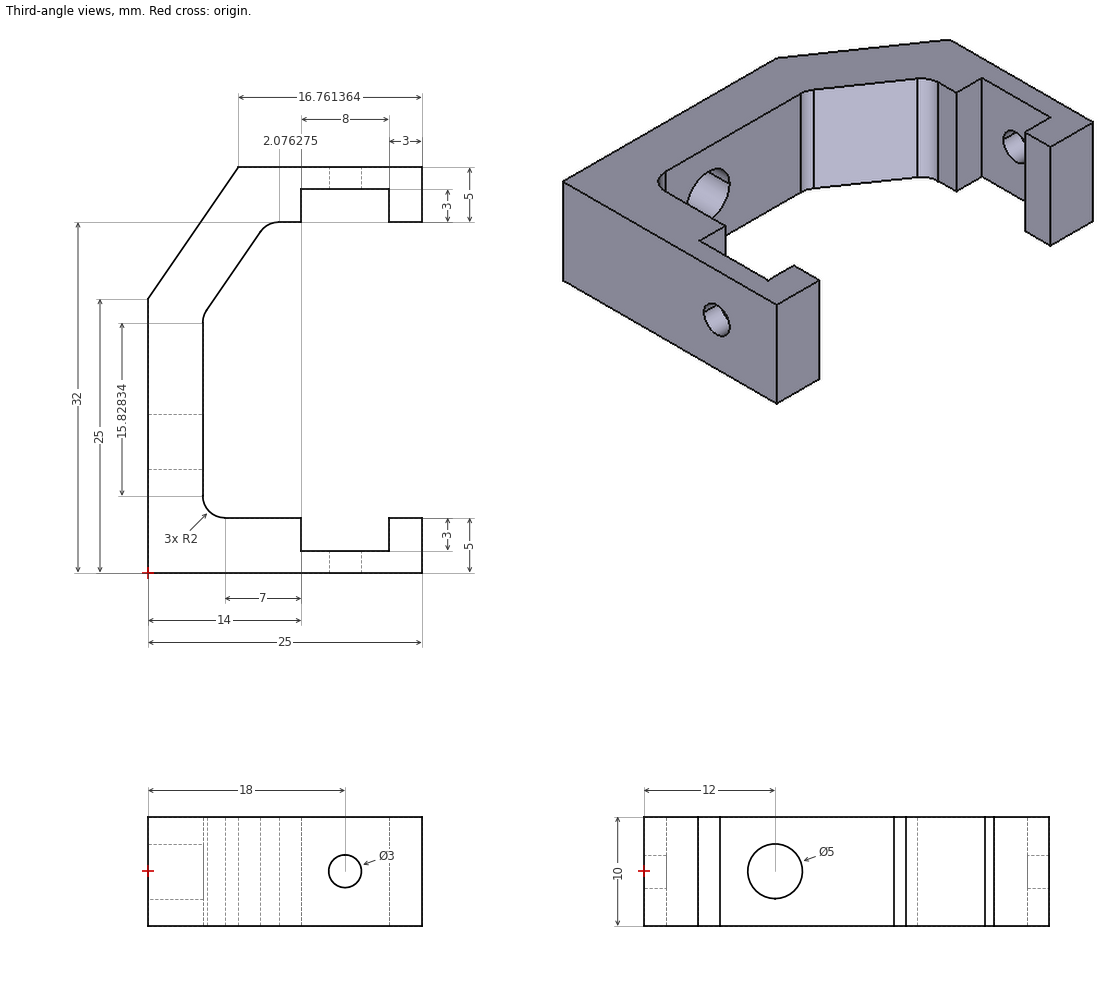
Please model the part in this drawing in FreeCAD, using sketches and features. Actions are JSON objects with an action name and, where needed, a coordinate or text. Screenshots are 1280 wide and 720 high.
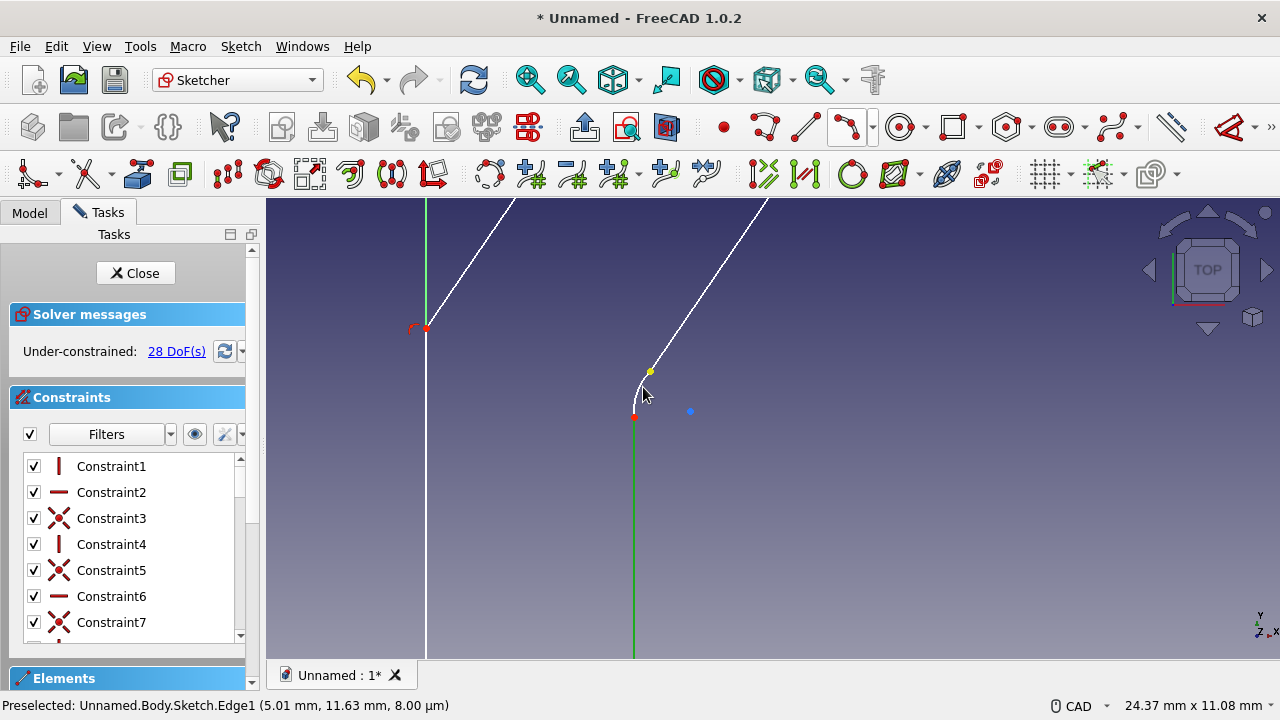
{"action": "left_click", "coordinate": [641, 384]}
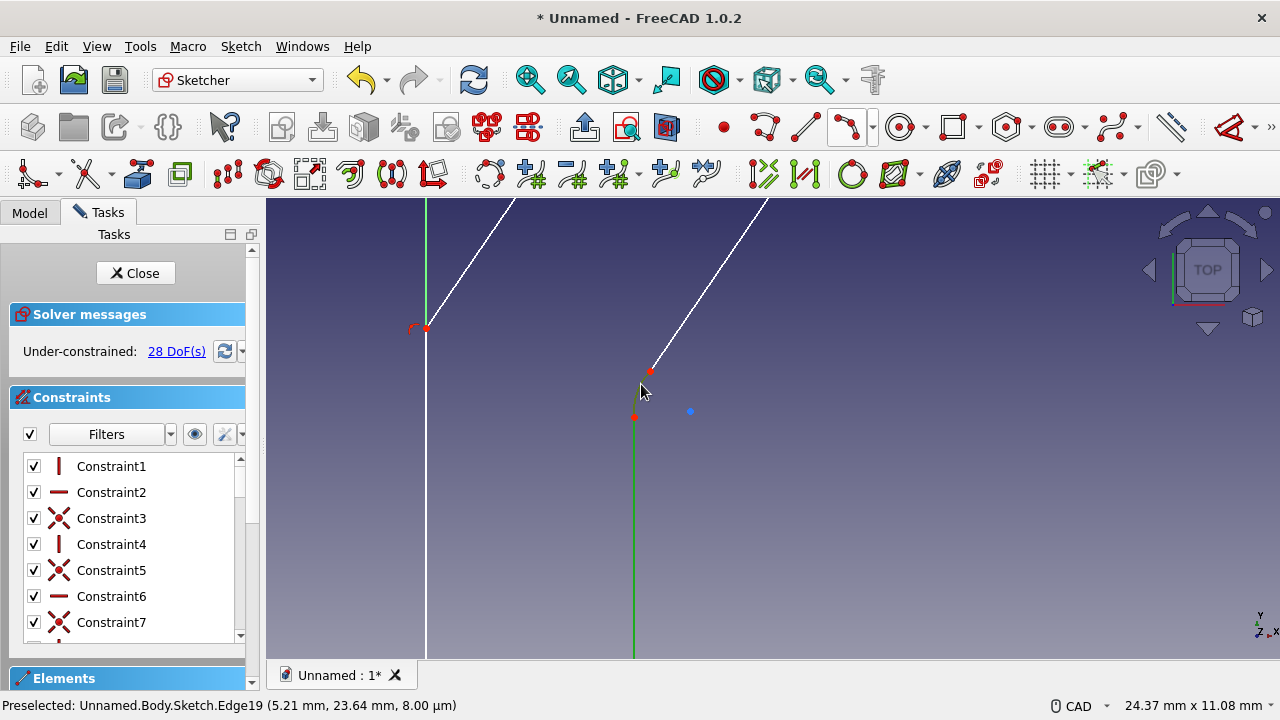
{"action": "key", "text": "t"}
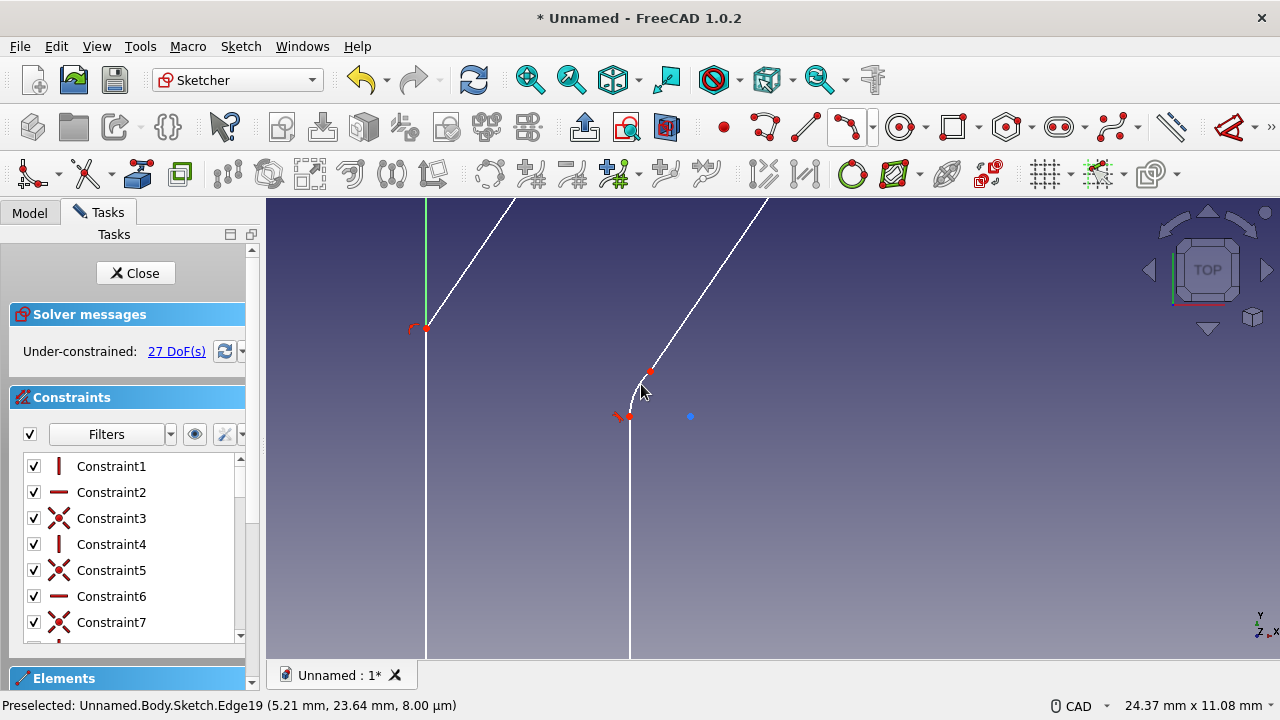
{"action": "scroll", "coordinate": [643, 386], "scroll_direction": "down", "scroll_amount": 8}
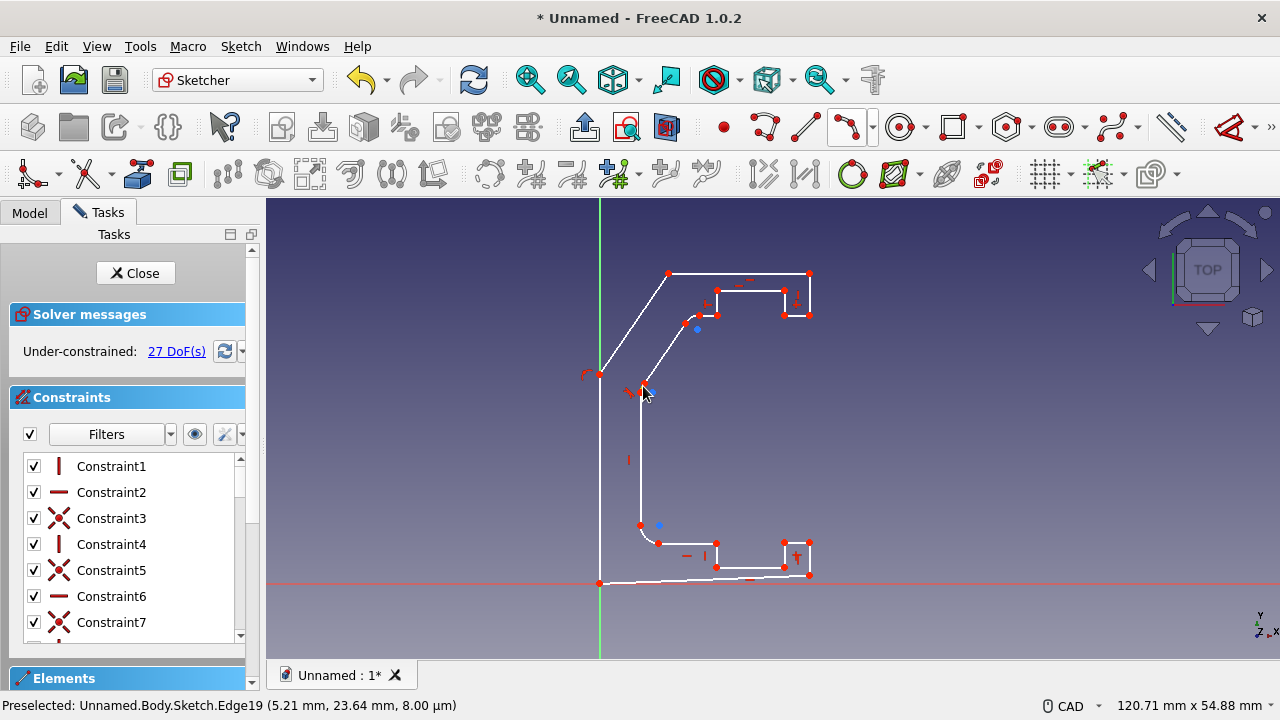
{"action": "left_click", "coordinate": [641, 433]}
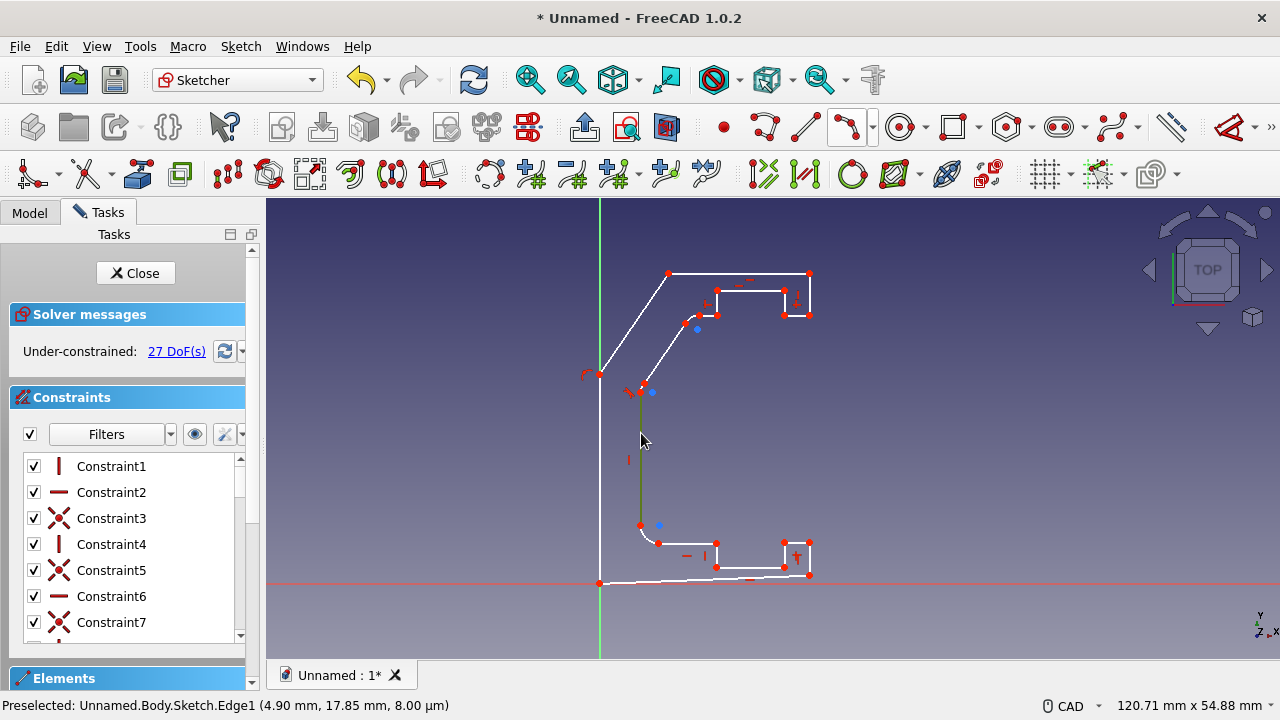
{"action": "left_click", "coordinate": [646, 538]}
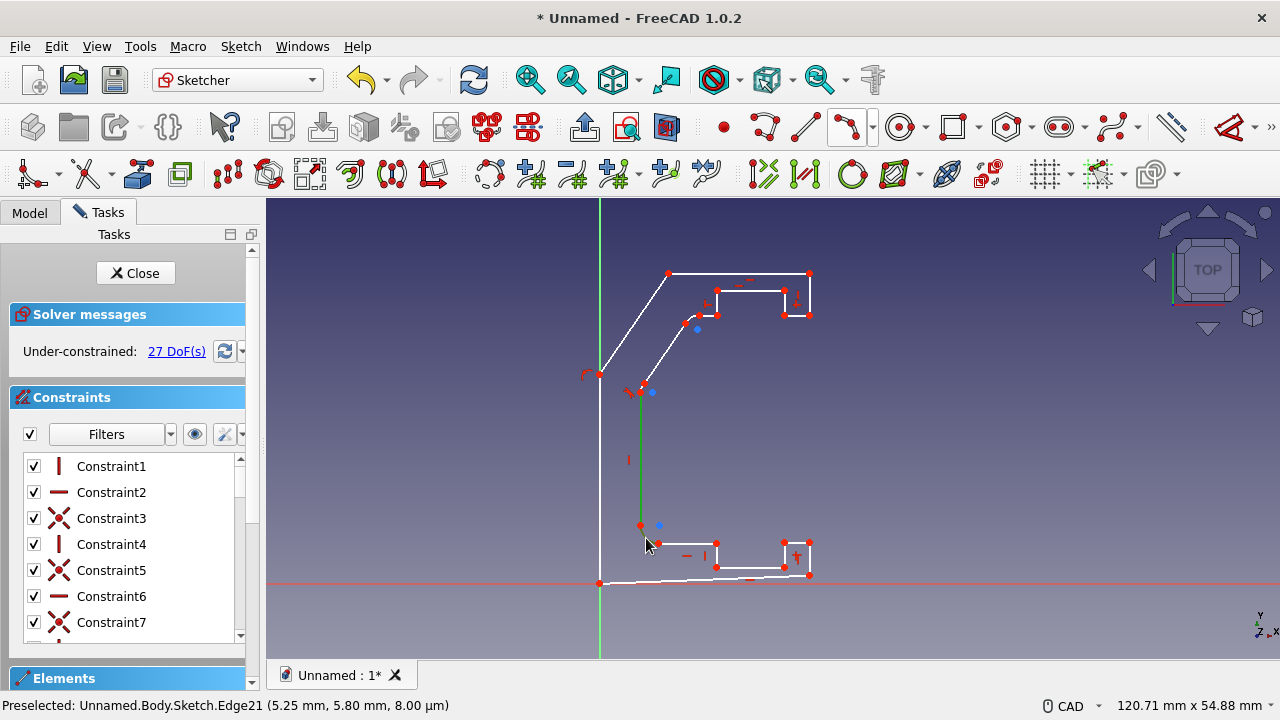
{"action": "key", "text": "t"}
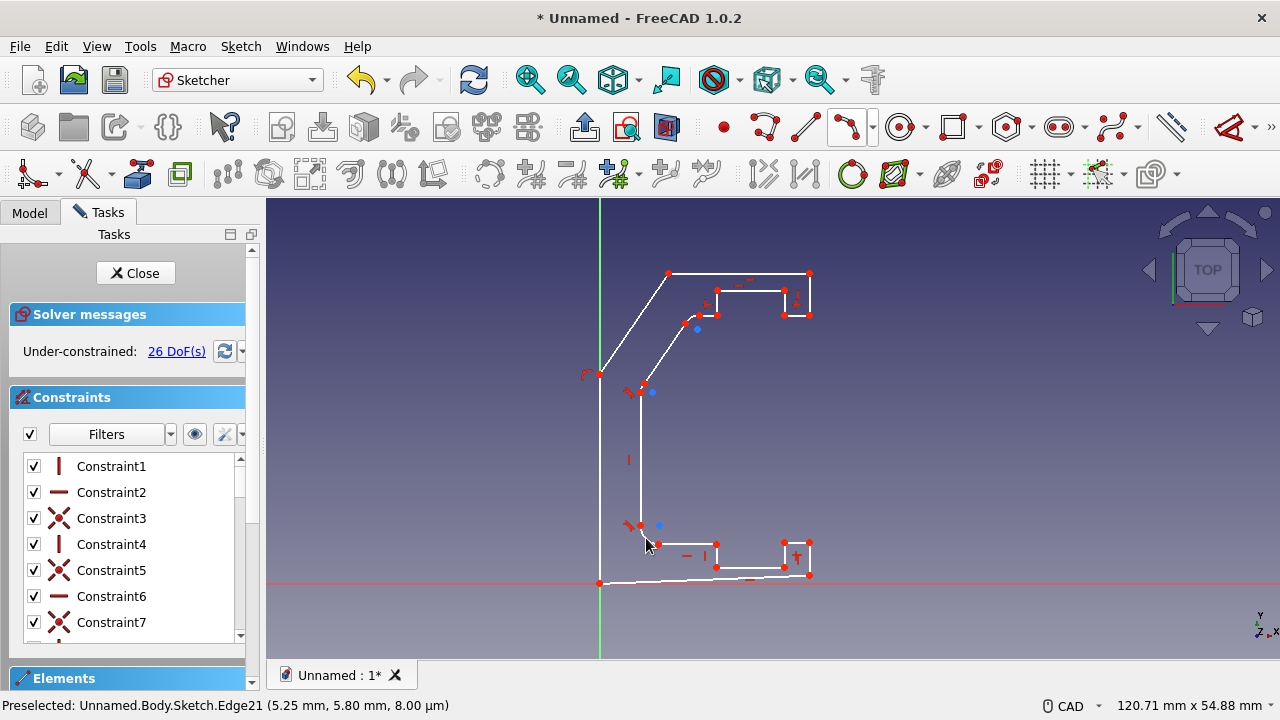
{"action": "left_click", "coordinate": [657, 365]}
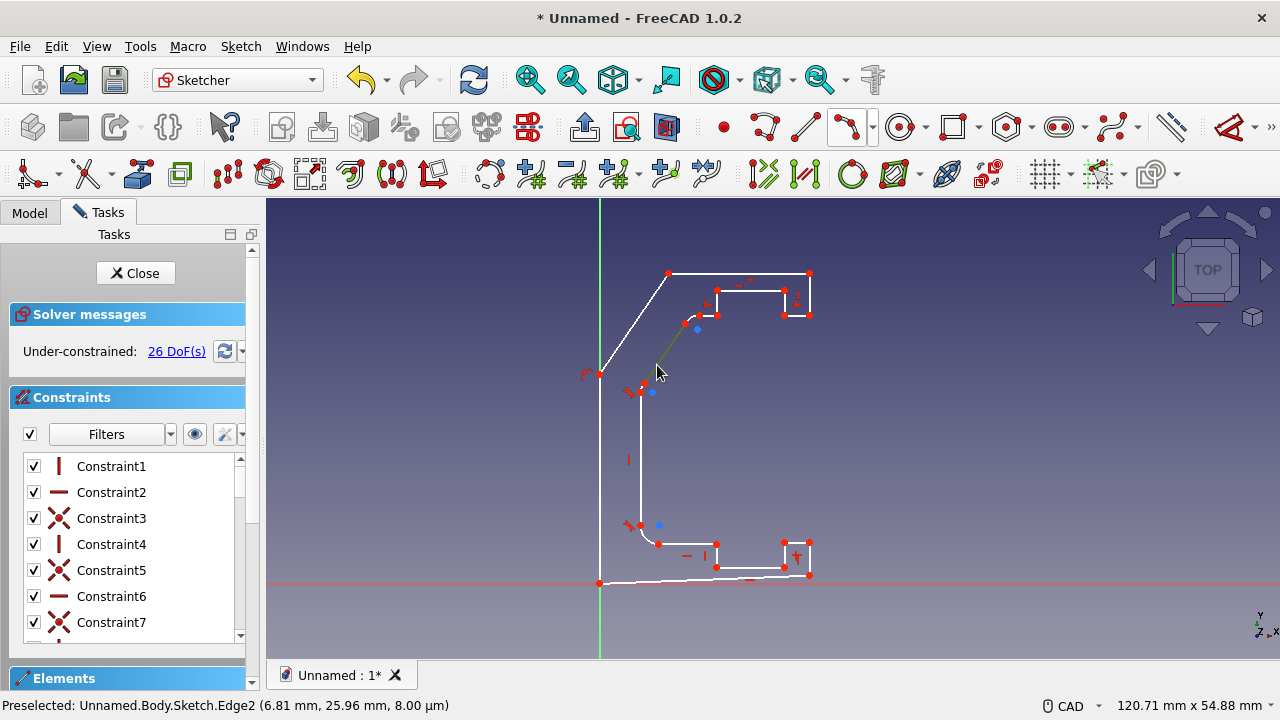
{"action": "scroll", "coordinate": [642, 388], "scroll_direction": "up", "scroll_amount": 5}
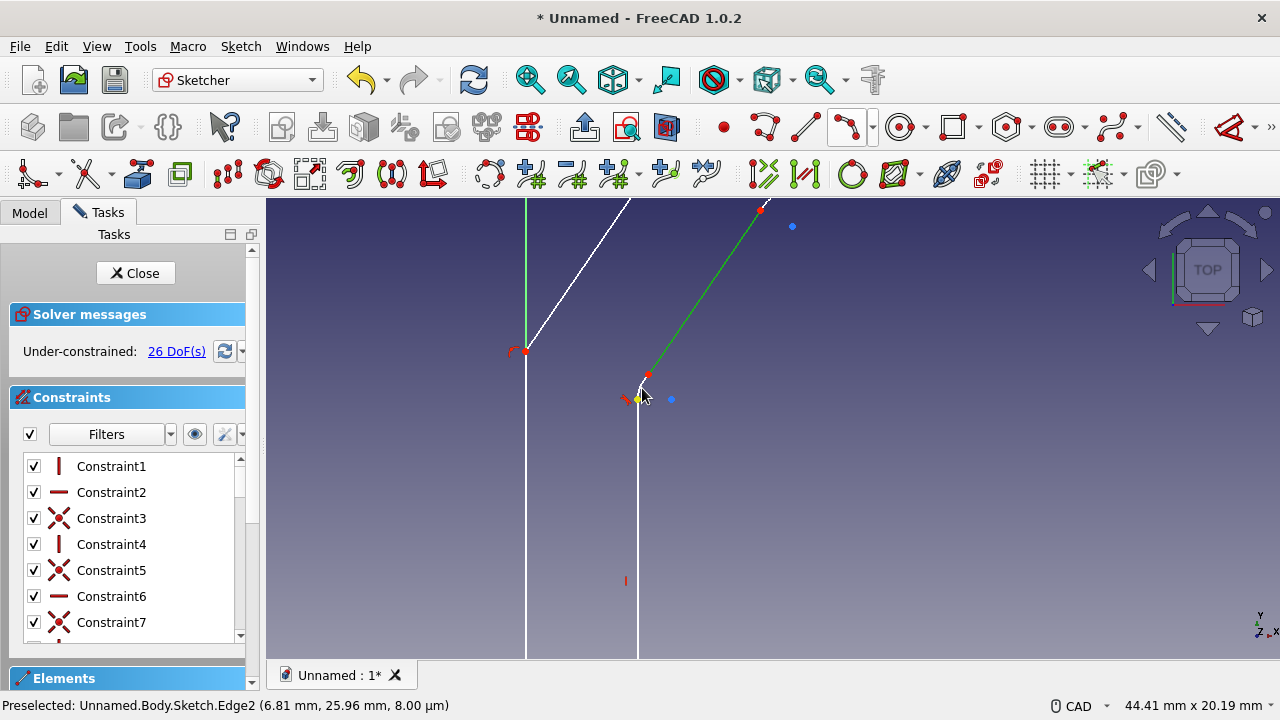
{"action": "left_click", "coordinate": [641, 386]}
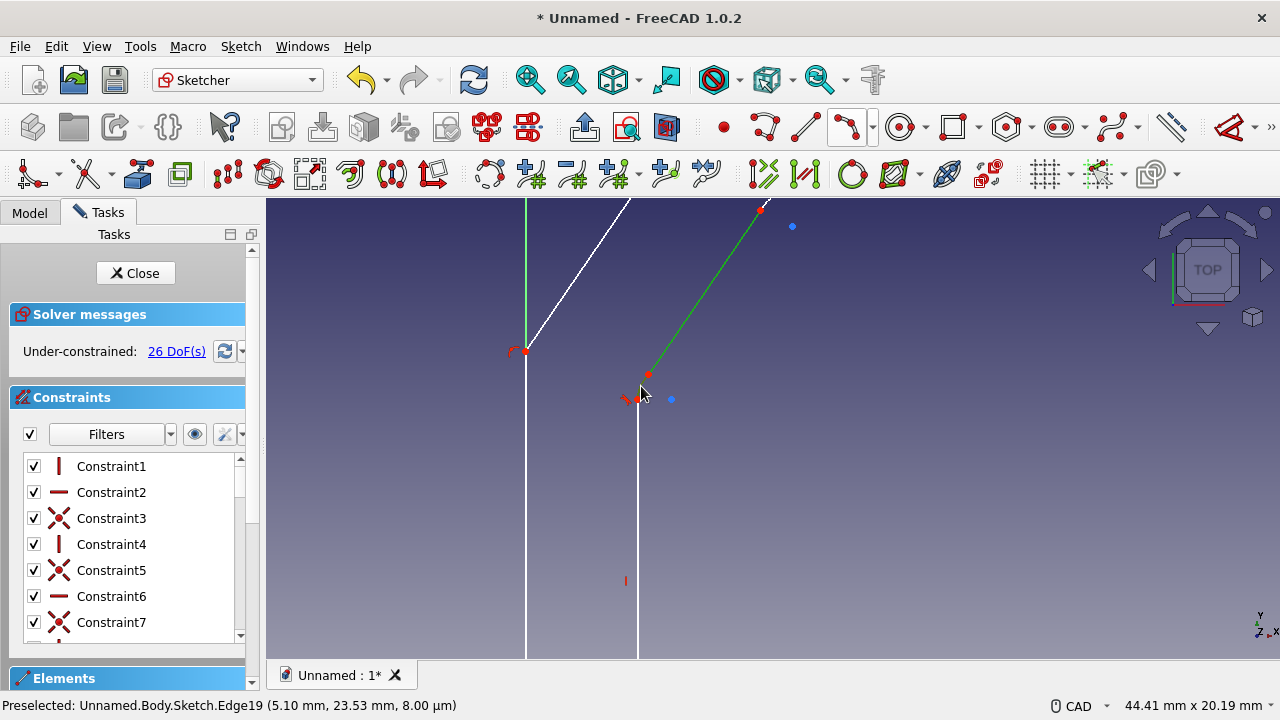
{"action": "key", "text": "t"}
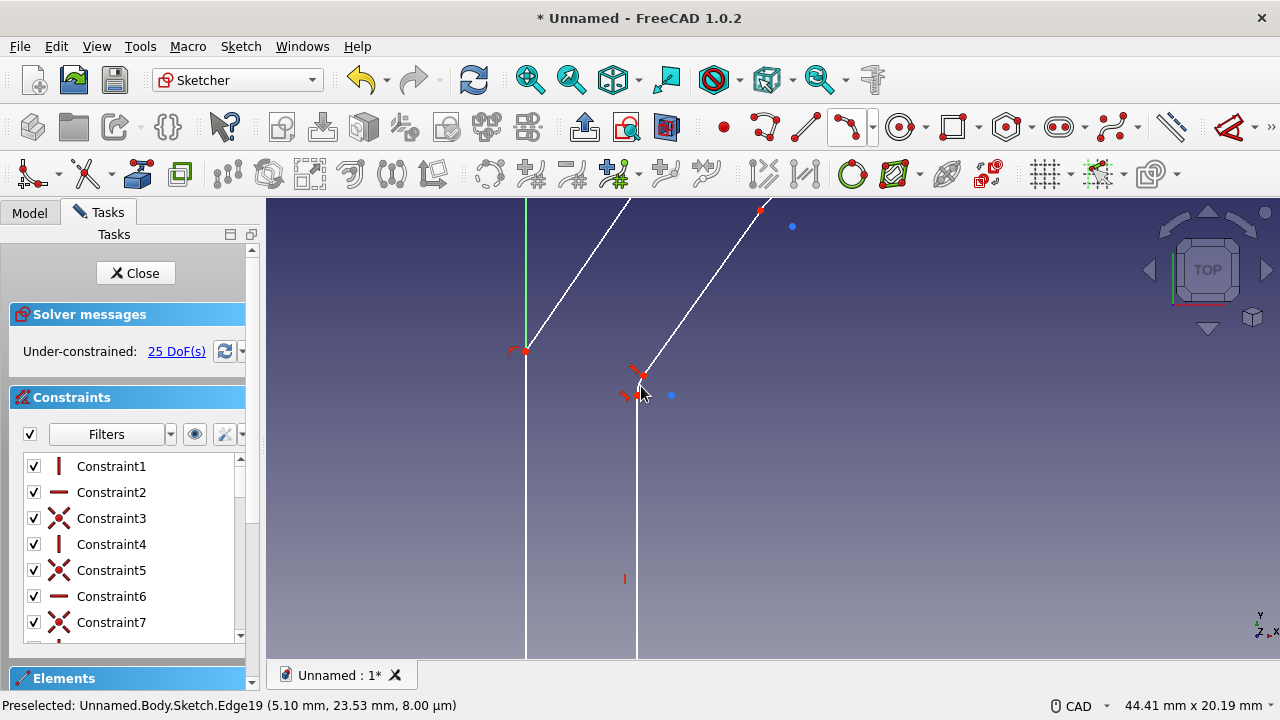
{"action": "left_click", "coordinate": [679, 326]}